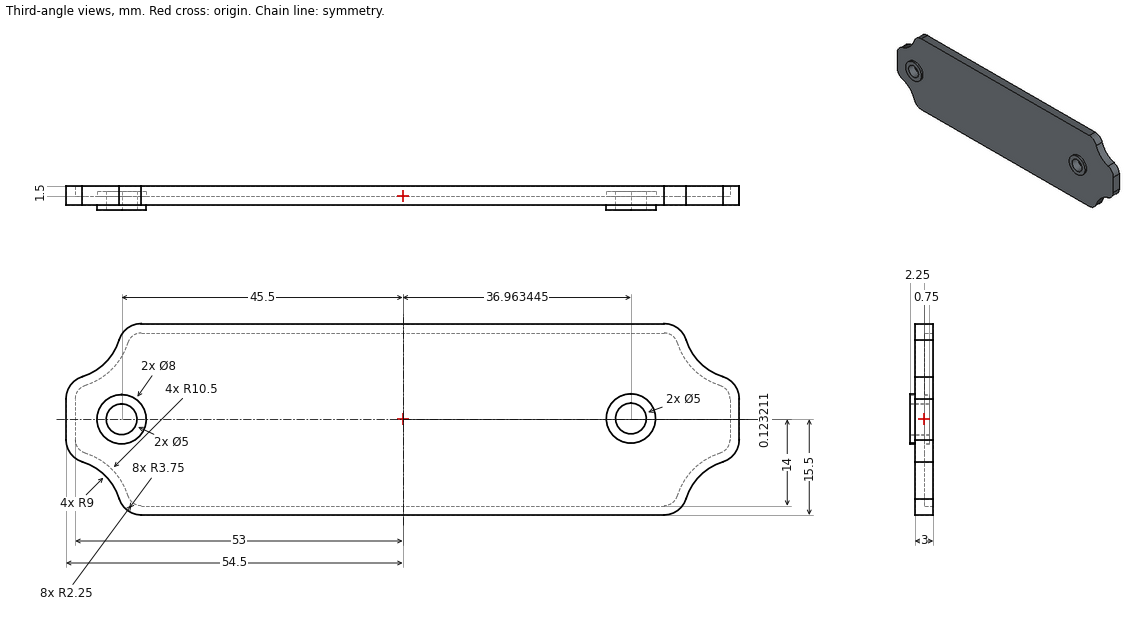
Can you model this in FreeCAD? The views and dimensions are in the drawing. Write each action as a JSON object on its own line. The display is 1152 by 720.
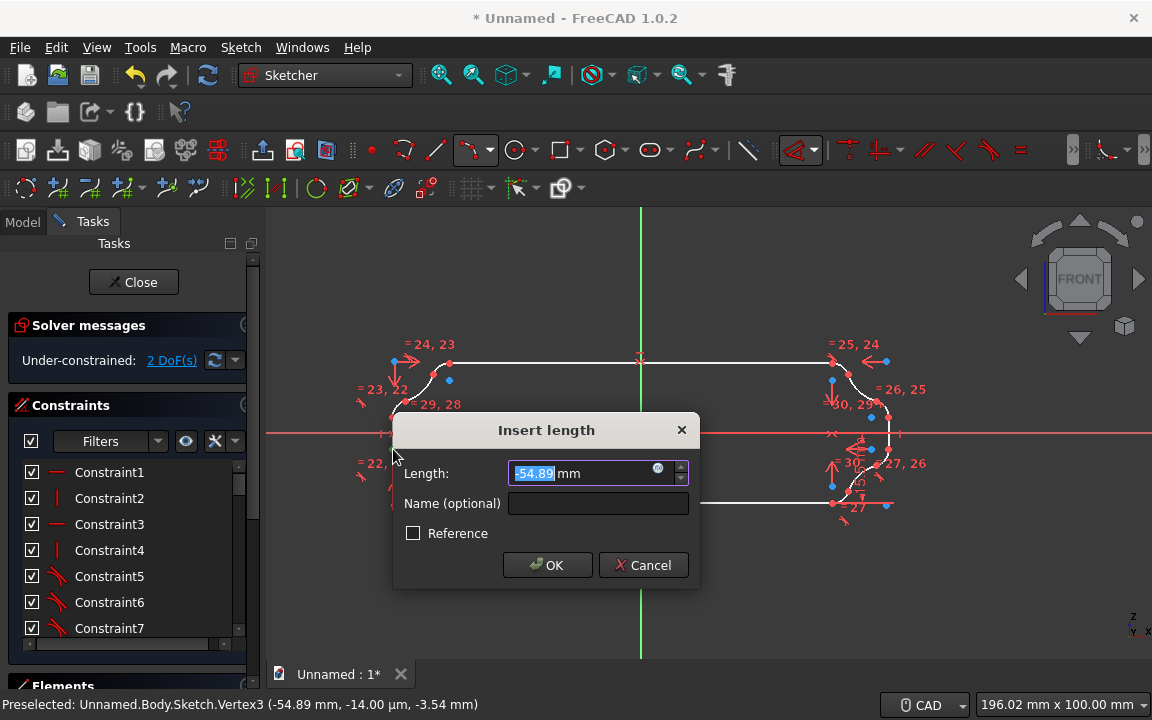
{"action": "type", "text": "-54.5"}
{"action": "key", "text": "Return"}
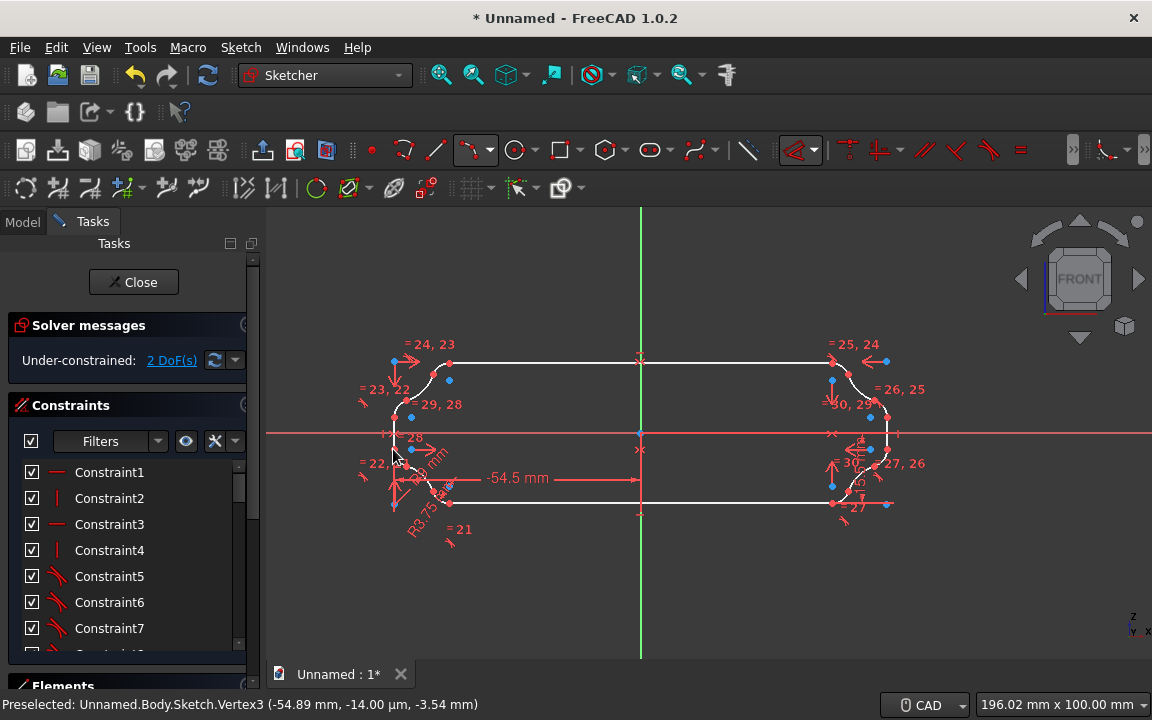
{"action": "left_click", "coordinate": [395, 505]}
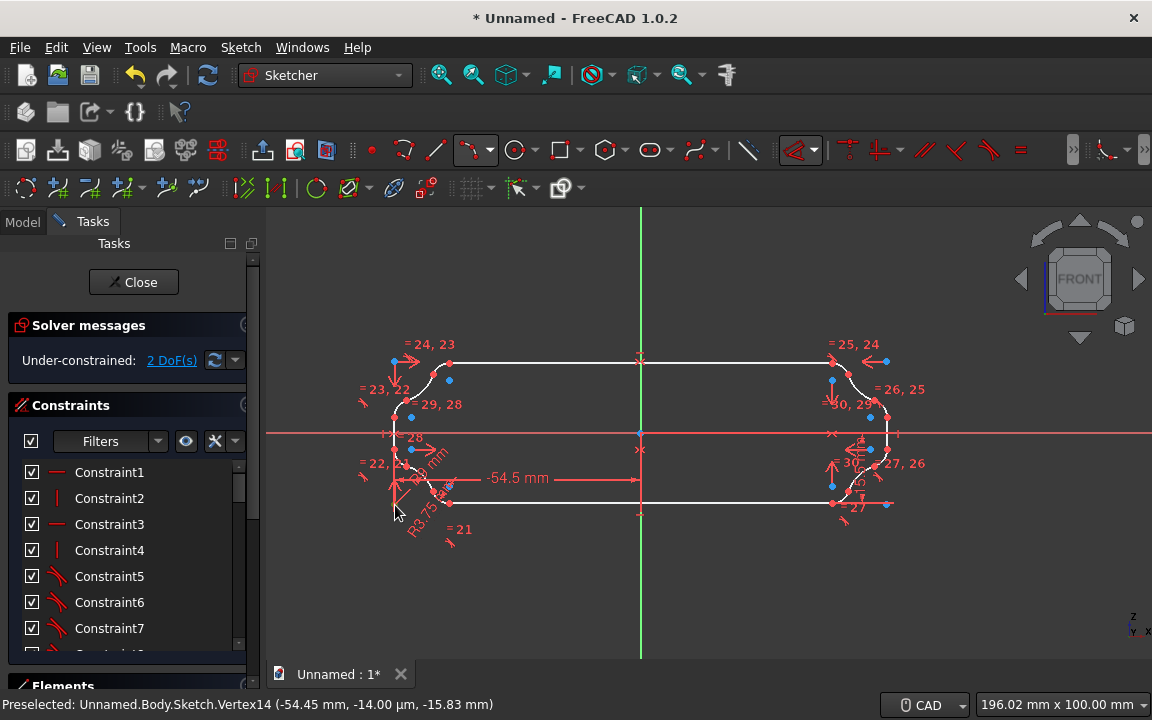
{"action": "key", "text": "l"}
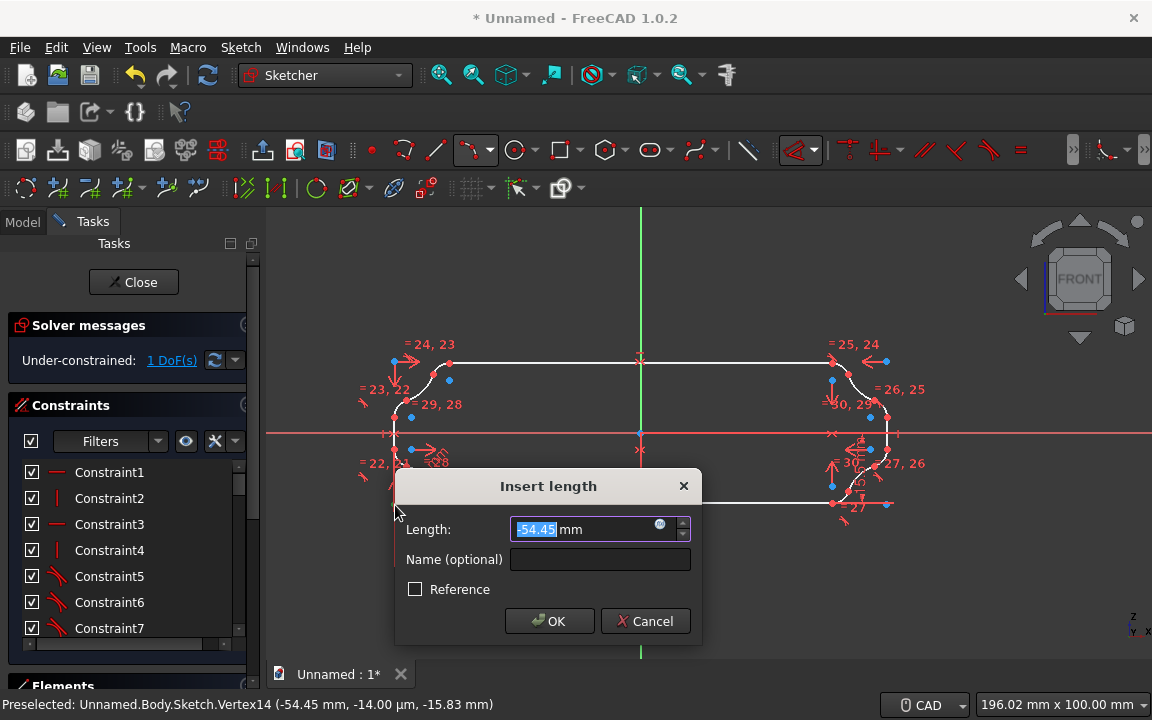
{"action": "type", "text": "-54.5"}
{"action": "key", "text": "Return"}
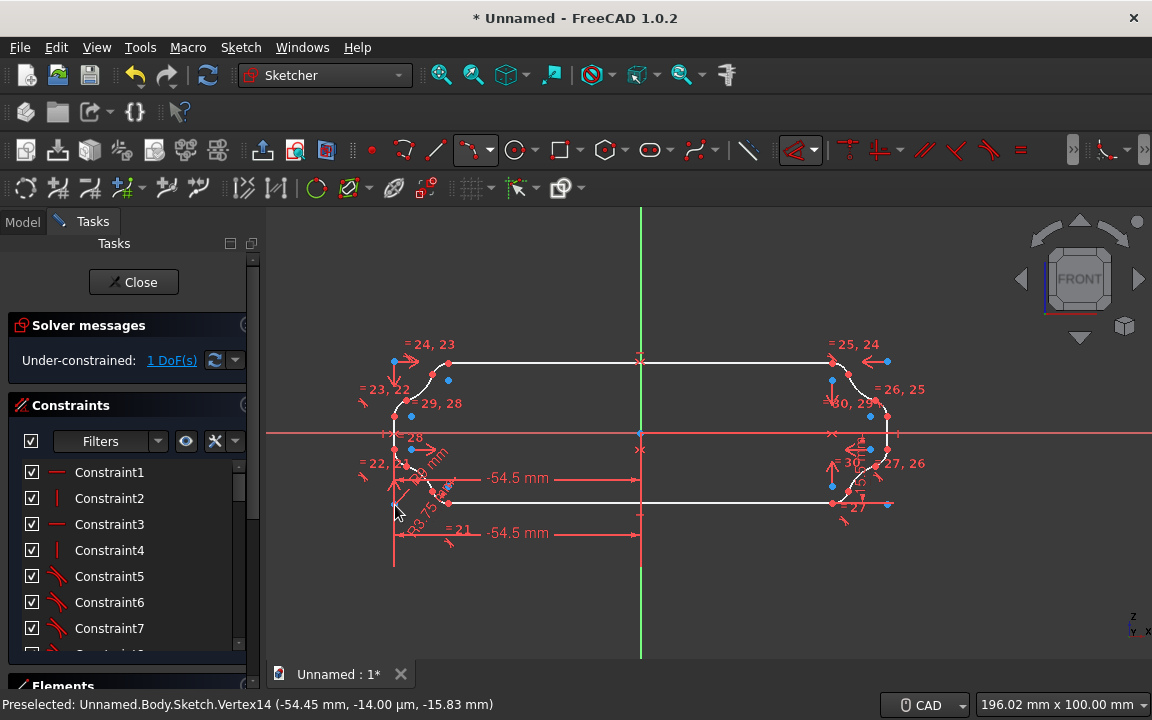
{"action": "left_click", "coordinate": [394, 505]}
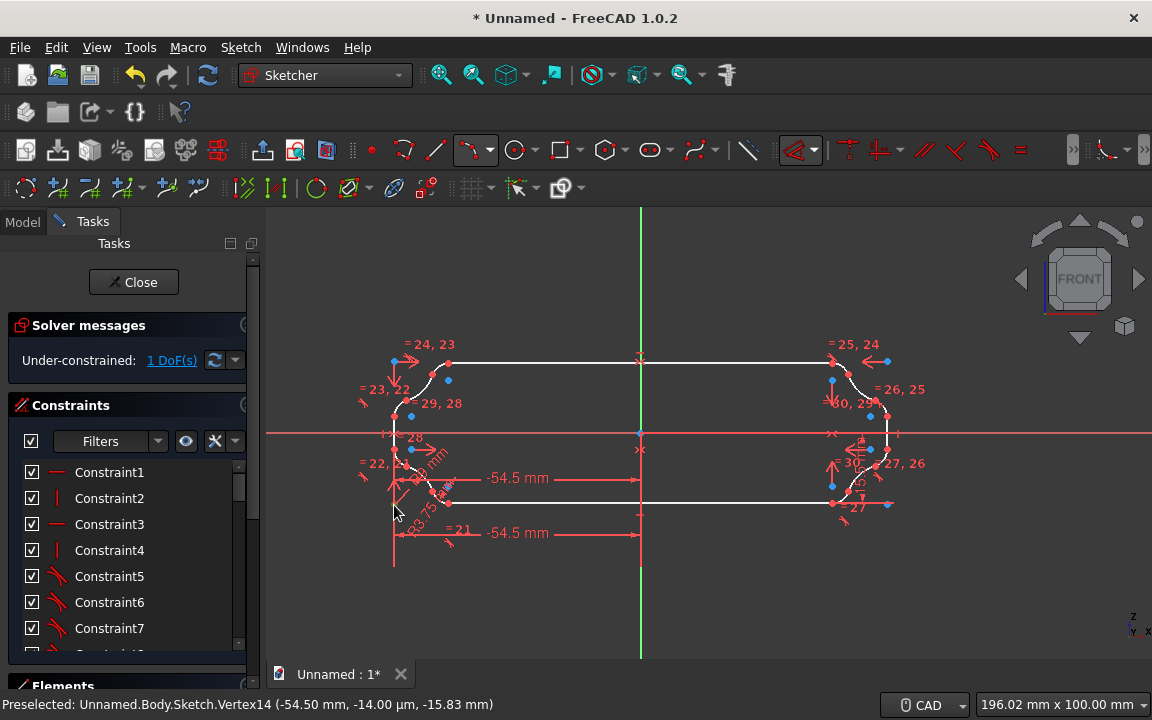
{"action": "left_click", "coordinate": [816, 150]}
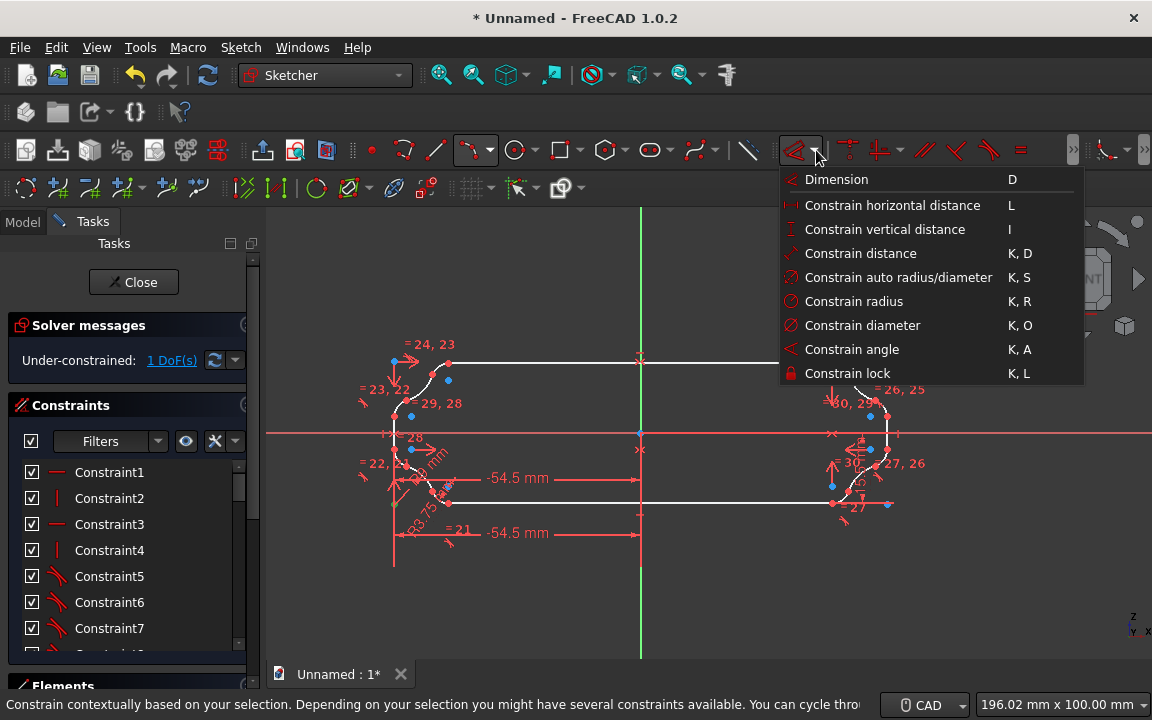
{"action": "left_click", "coordinate": [932, 229]}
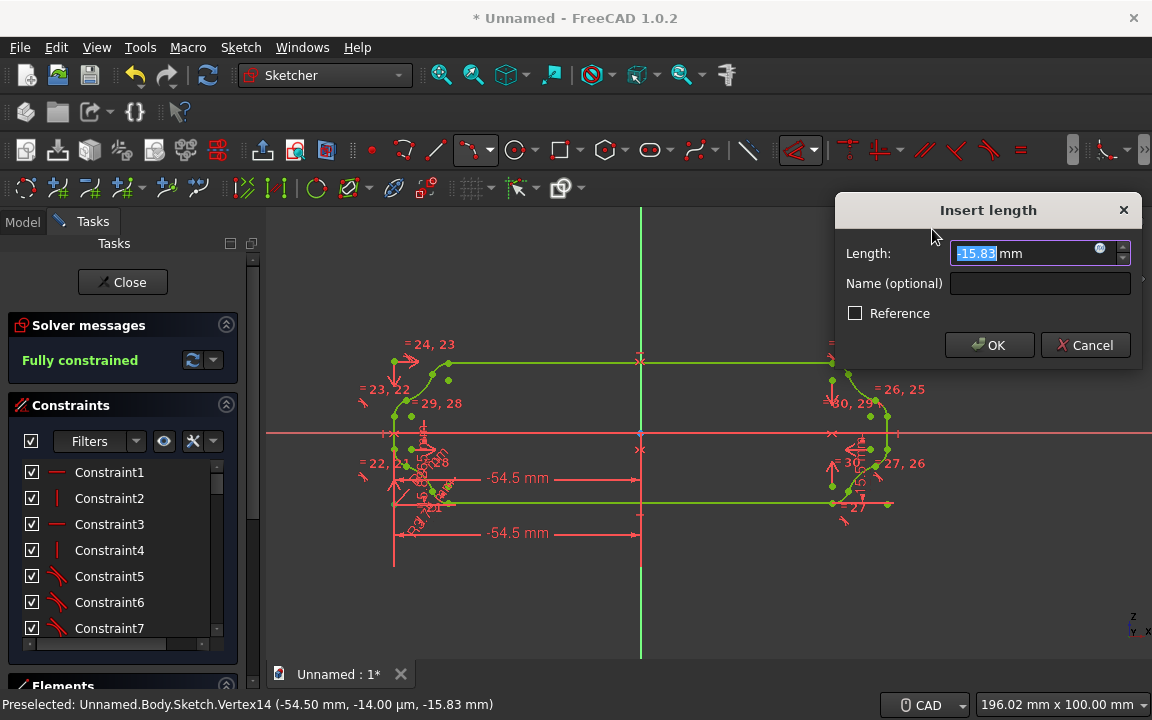
{"action": "type", "text": "-15.5"}
{"action": "key", "text": "Return"}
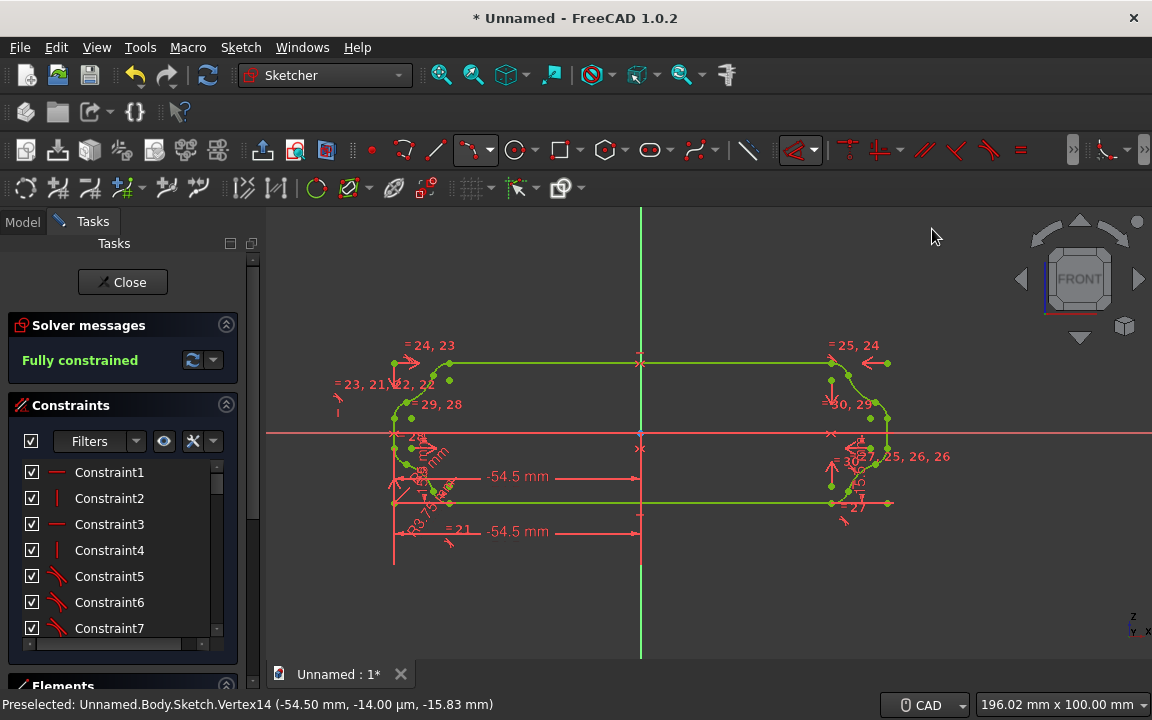
{"action": "left_click", "coordinate": [123, 282]}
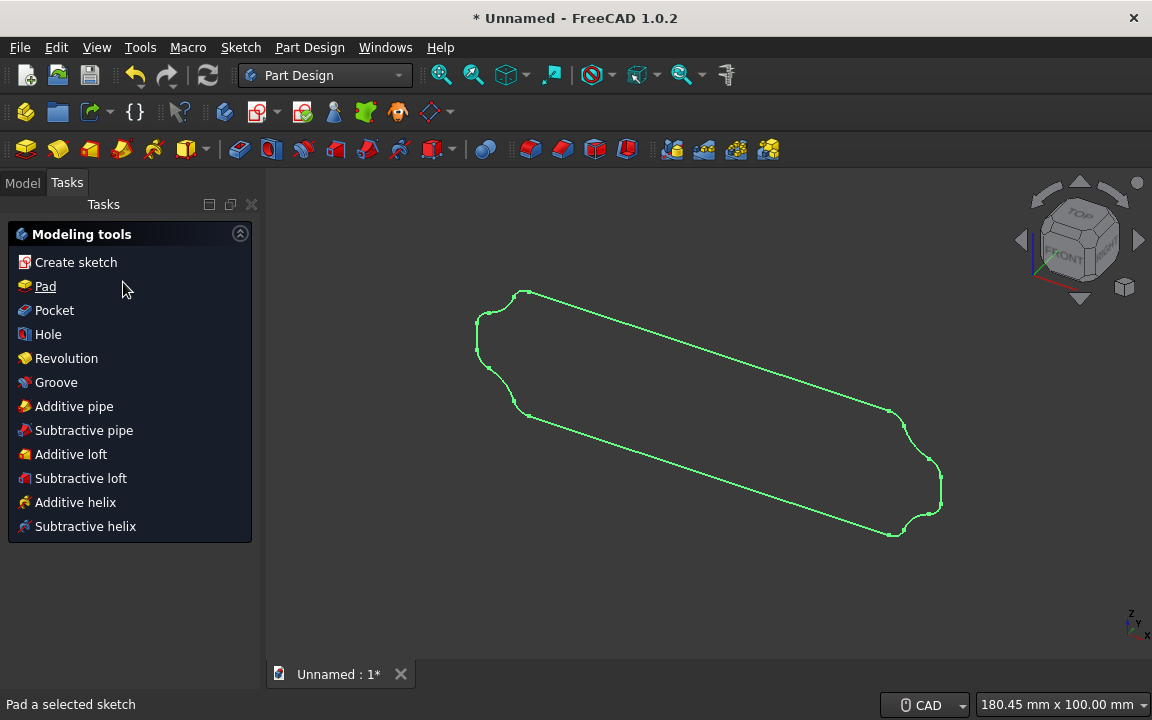
{"action": "left_click", "coordinate": [26, 150]}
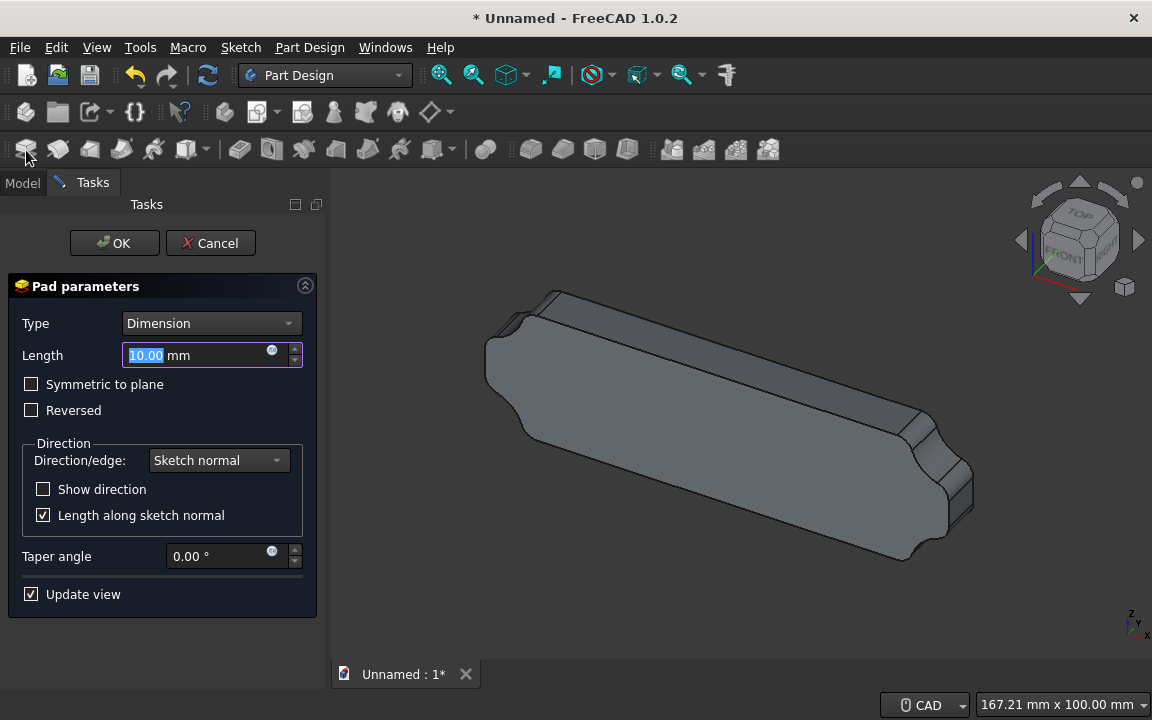
{"action": "type", "text": "3"}
{"action": "key", "text": "Tab"}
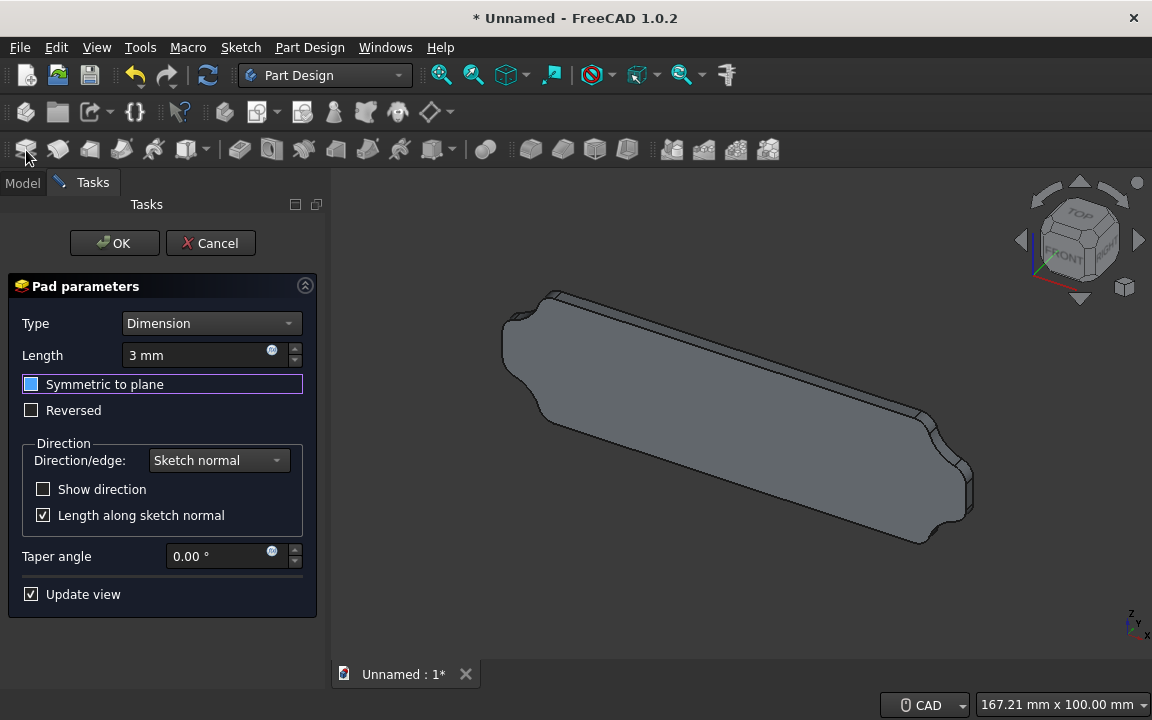
{"action": "left_click", "coordinate": [30, 384]}